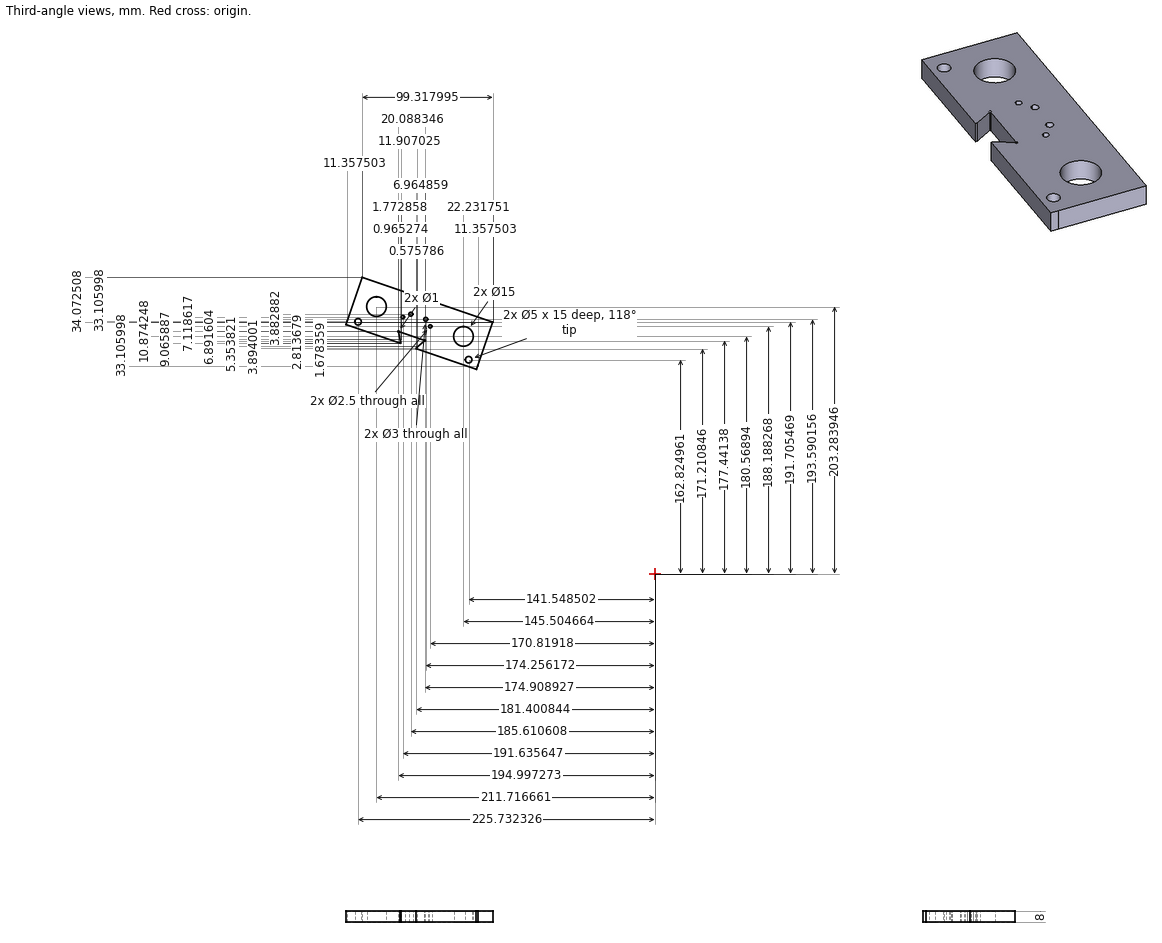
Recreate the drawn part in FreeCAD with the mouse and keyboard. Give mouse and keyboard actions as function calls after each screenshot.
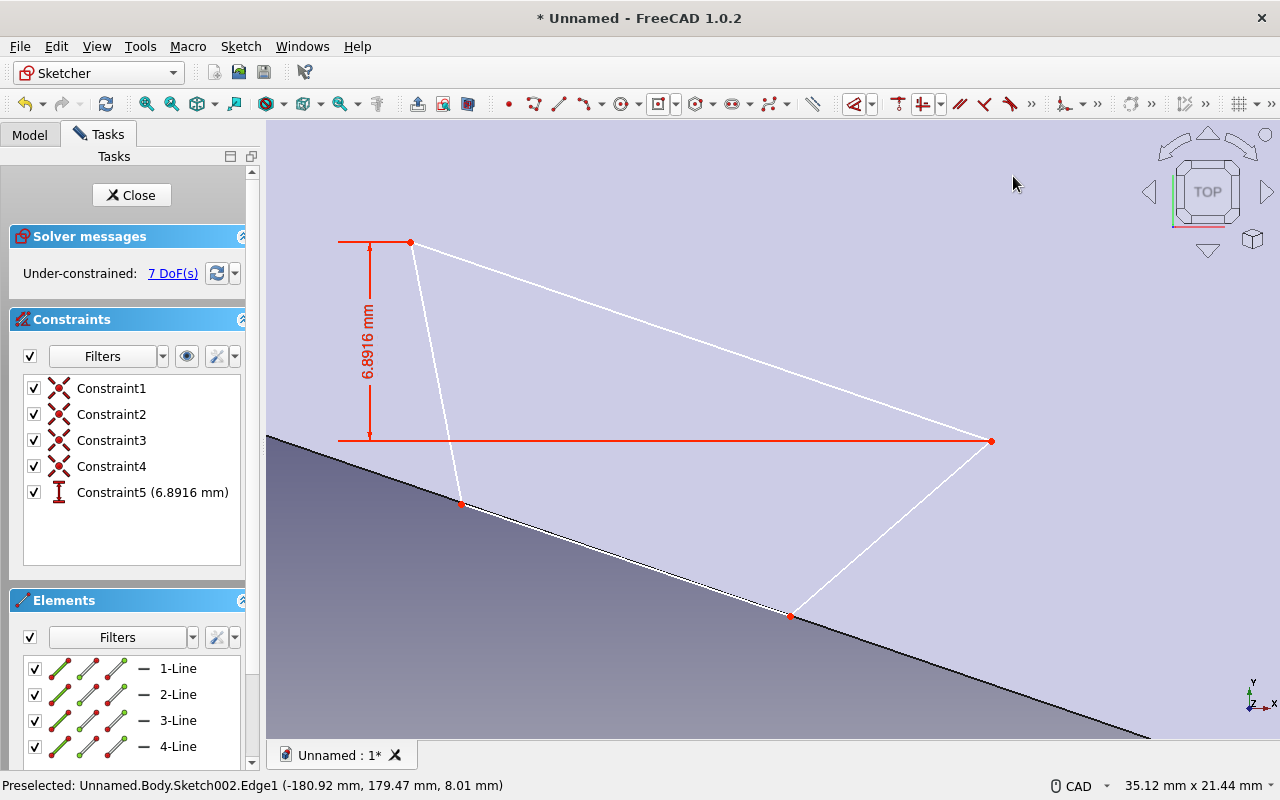
click(426, 321)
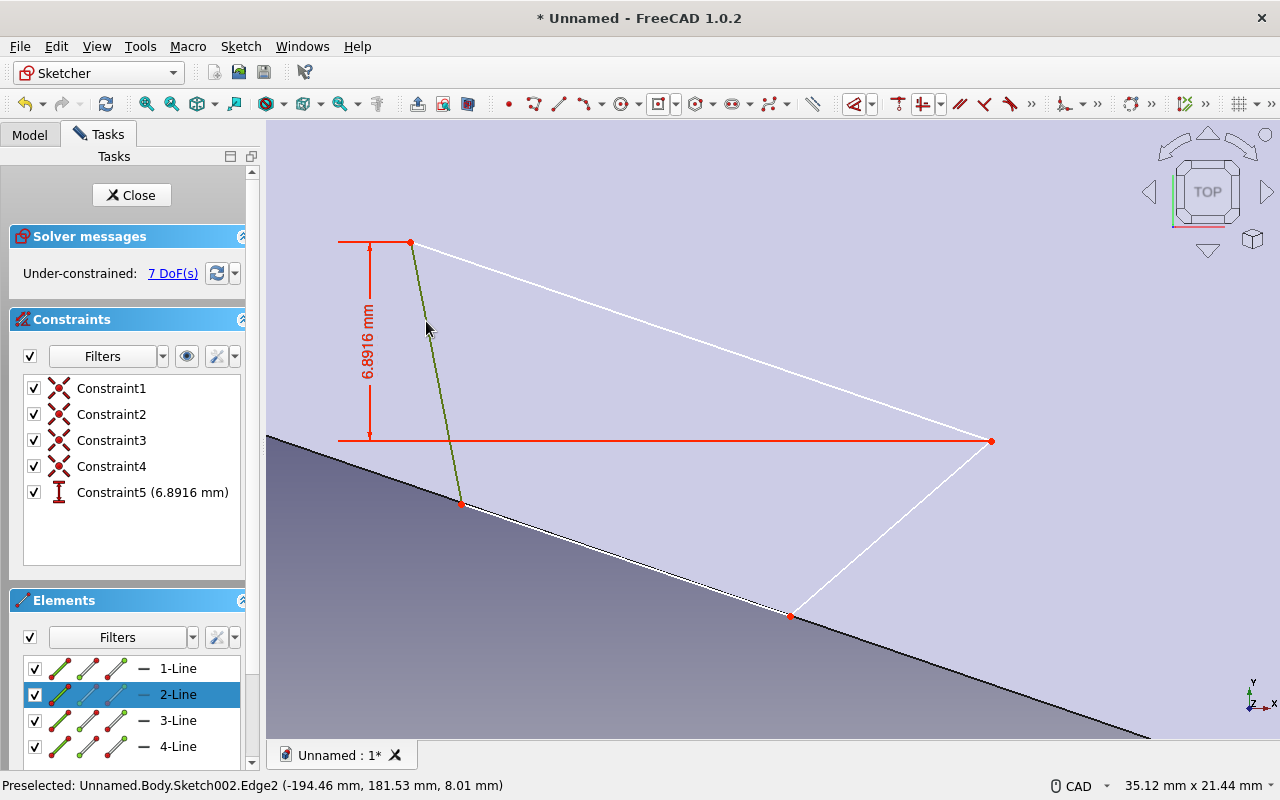
key(l)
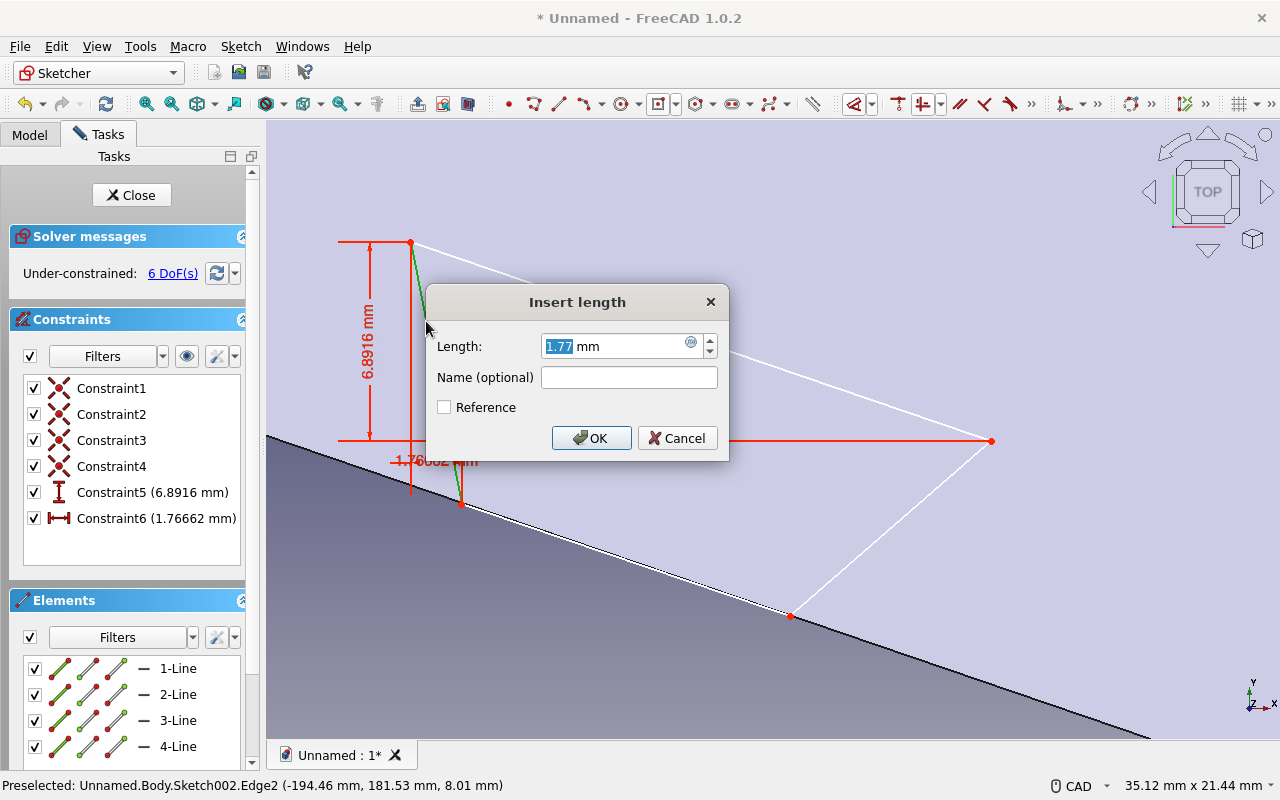
text(1.772858)
key(Return)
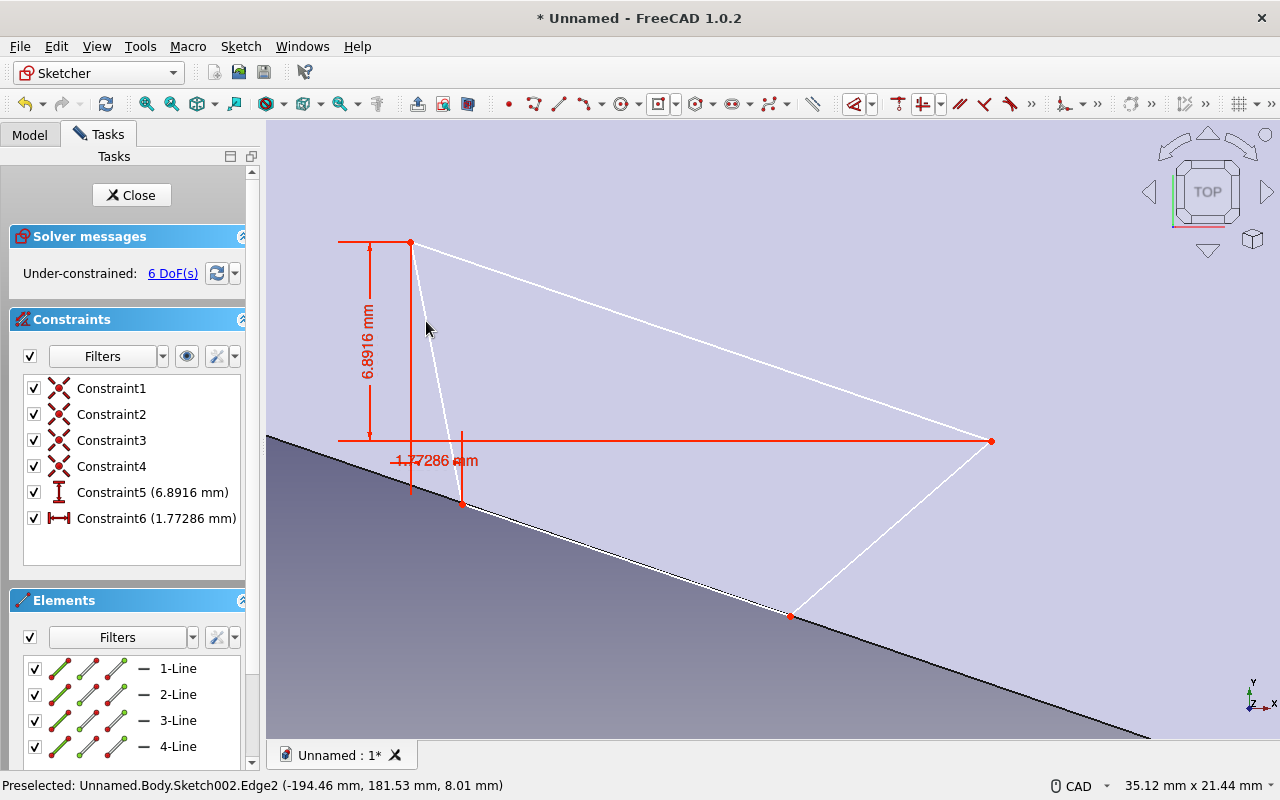
click(426, 321)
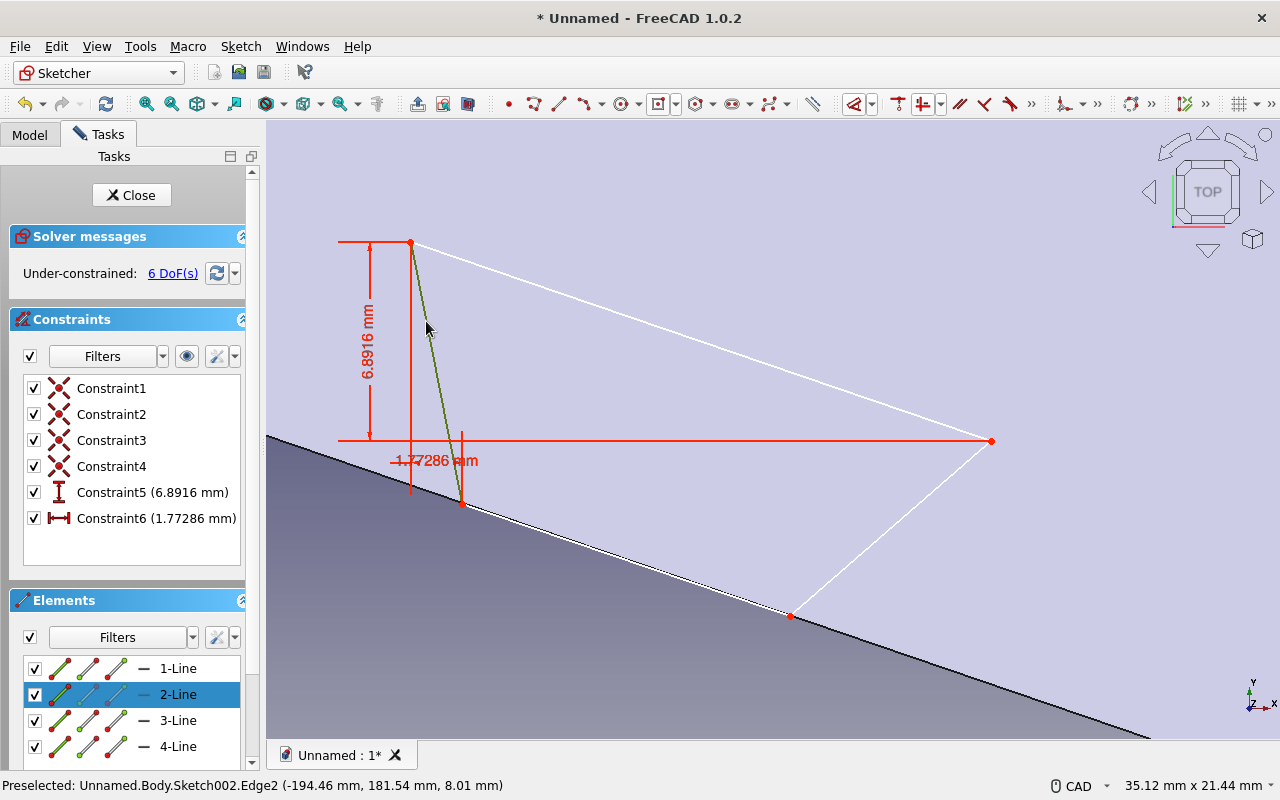
click(872, 104)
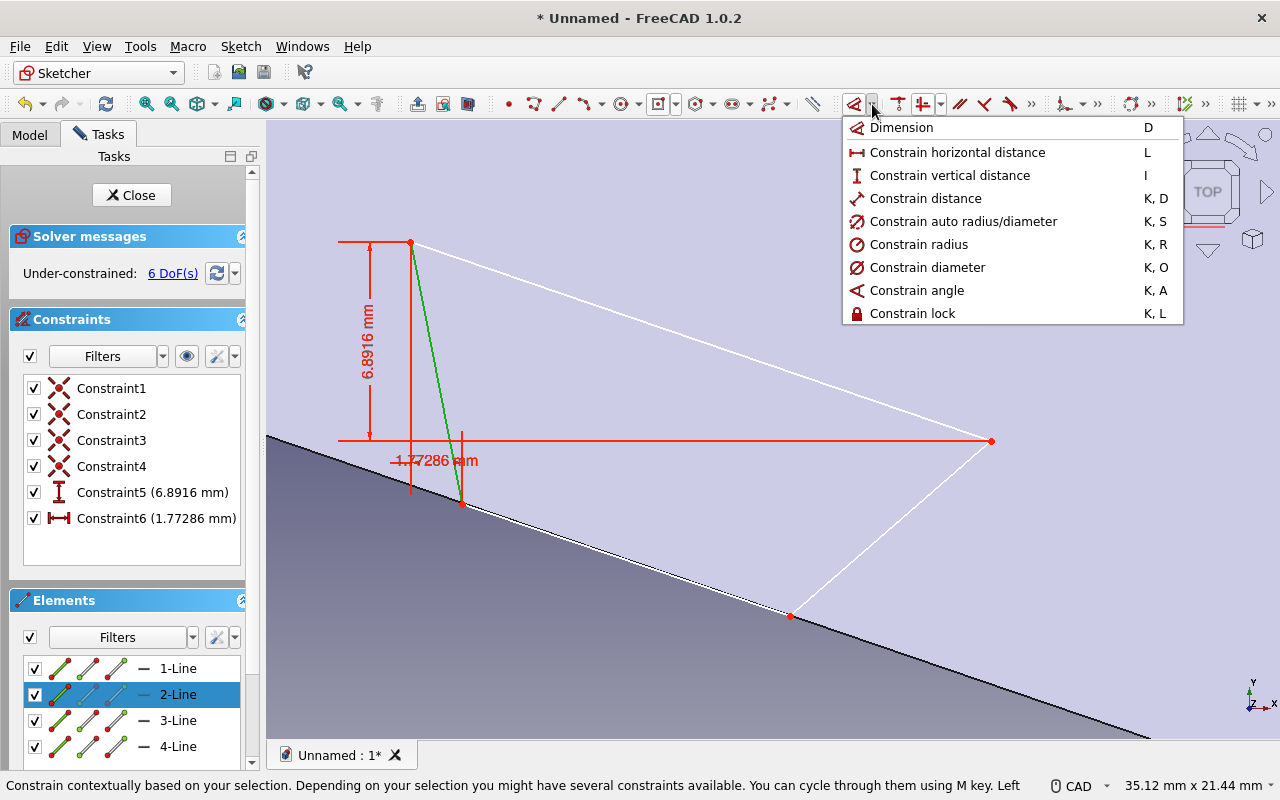
click(1013, 176)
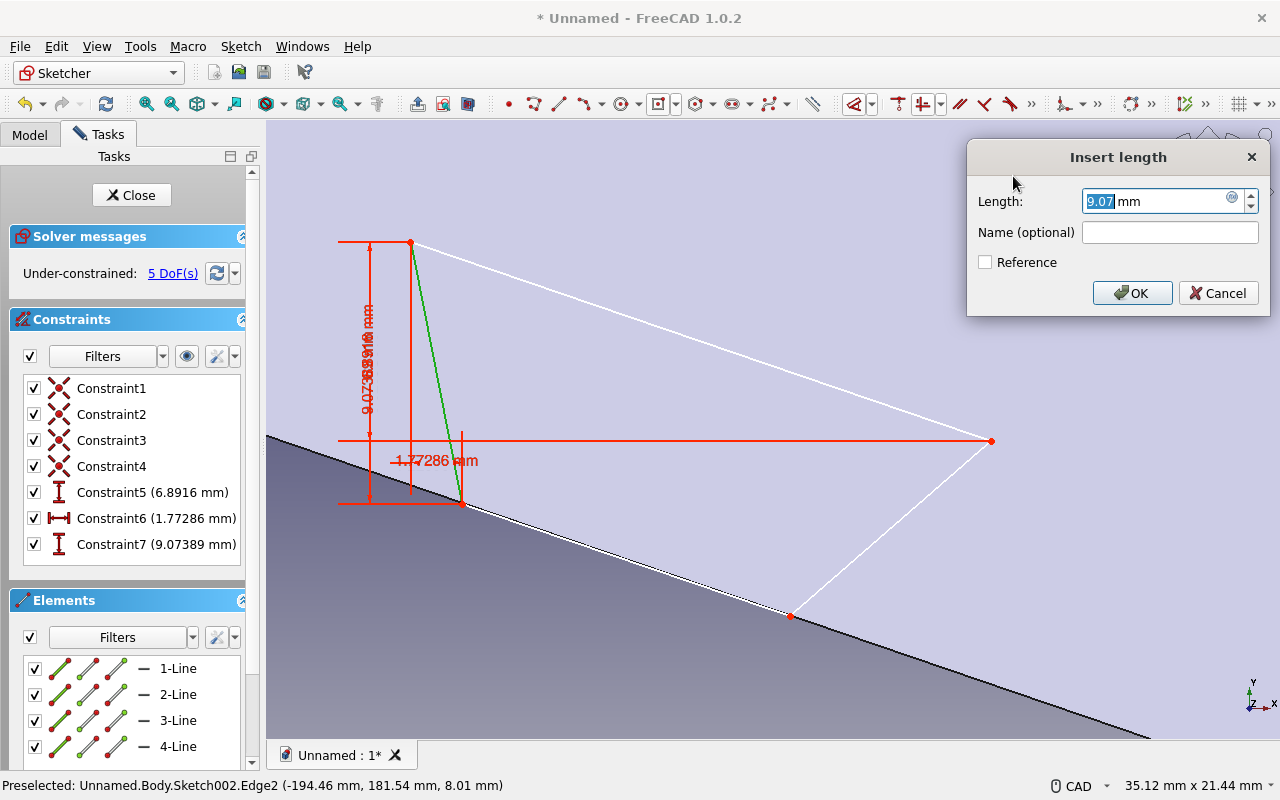
text(9.065887)
key(Return)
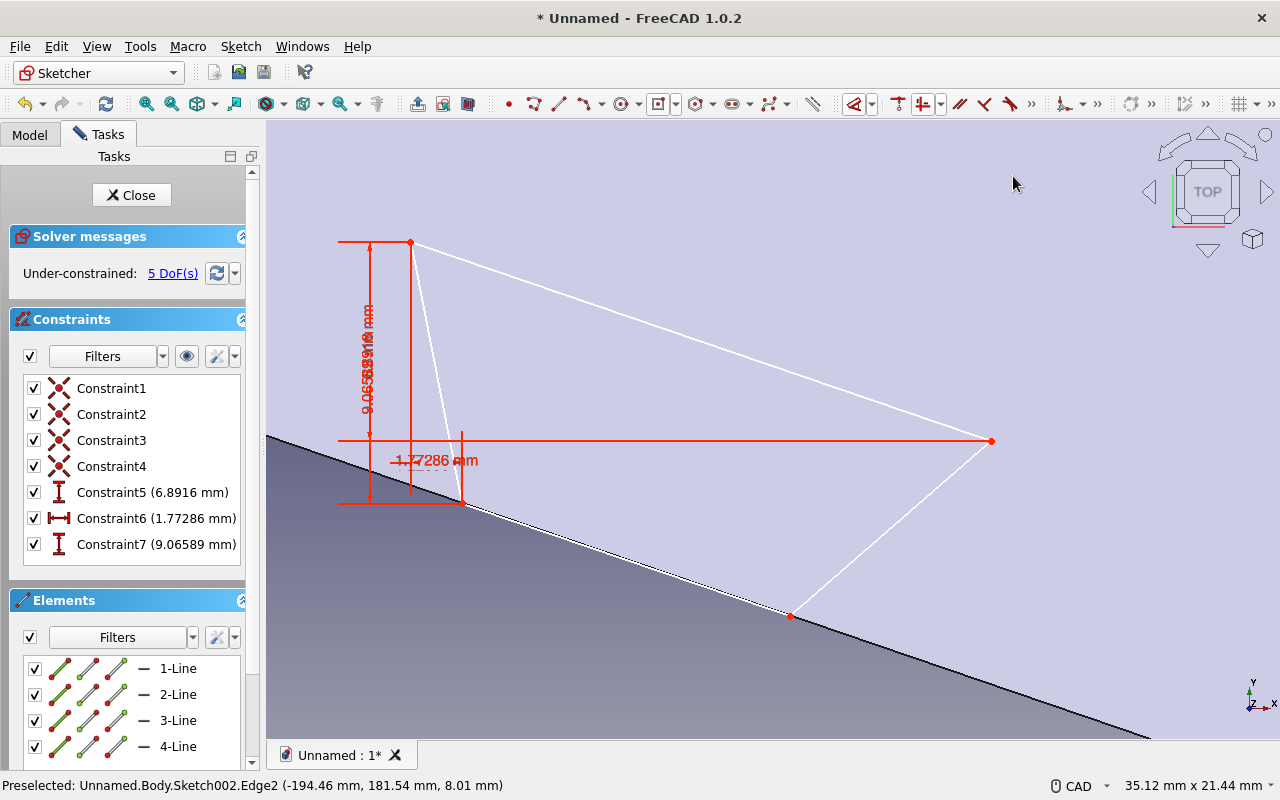
click(561, 537)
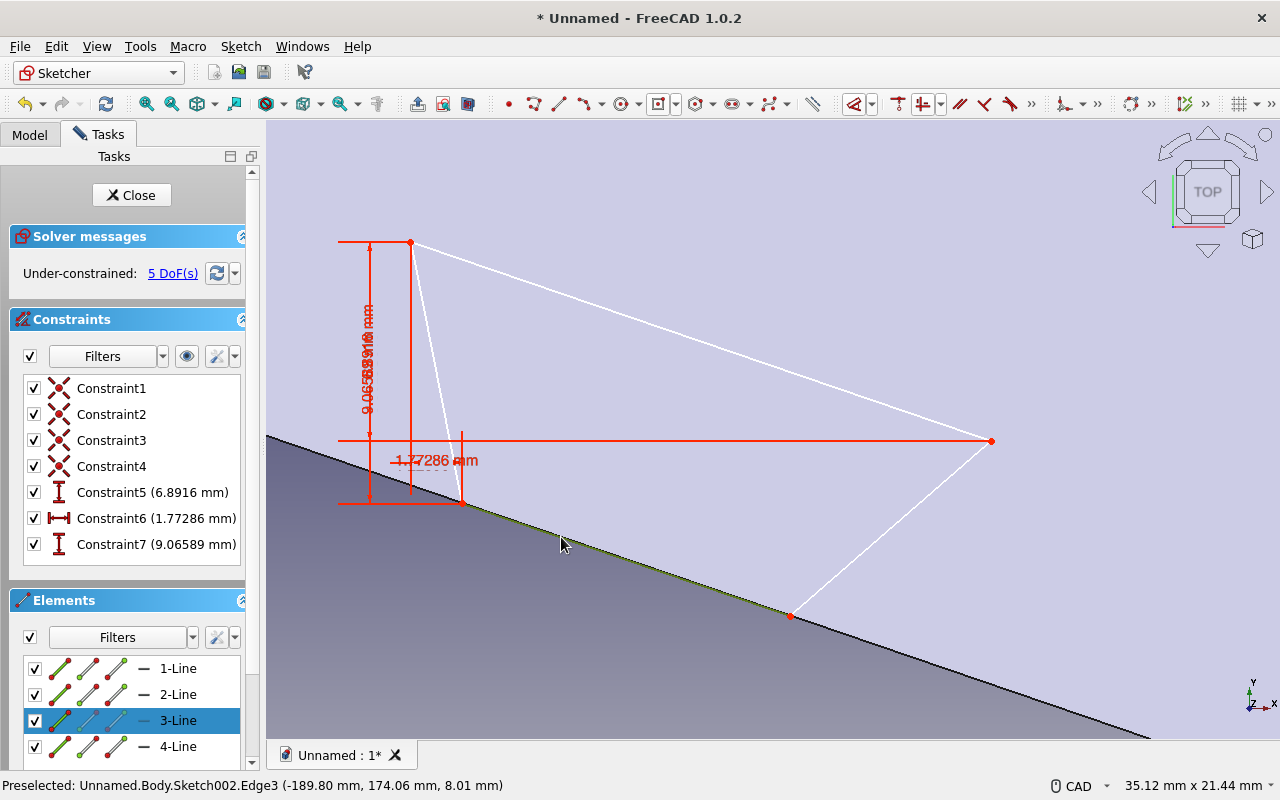
key(i)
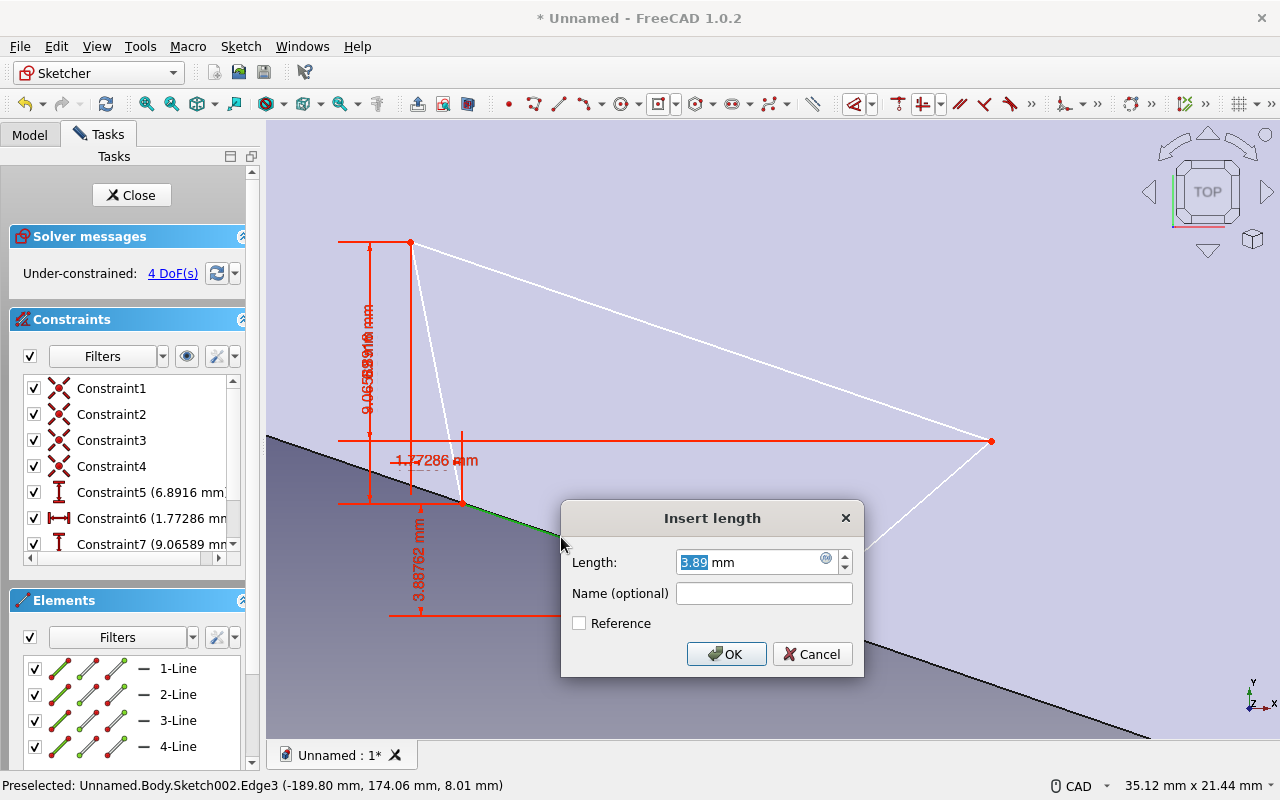
text(3.894001)
key(Return)